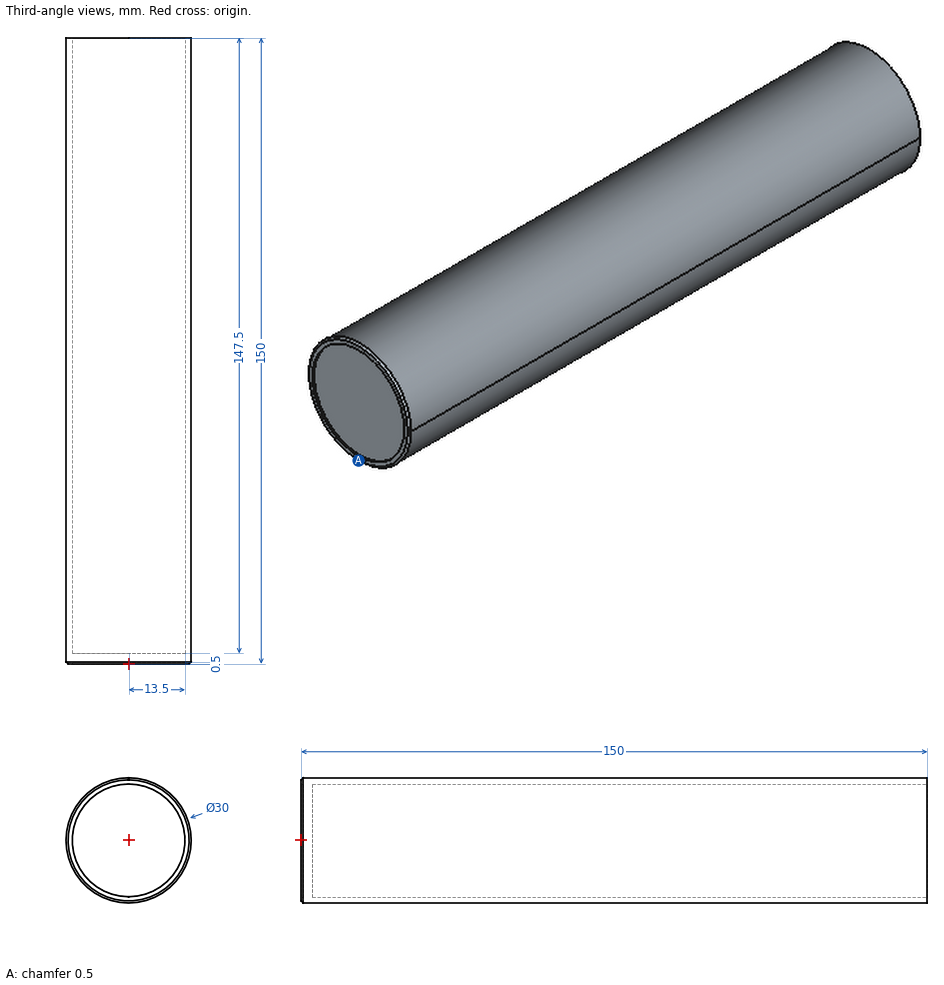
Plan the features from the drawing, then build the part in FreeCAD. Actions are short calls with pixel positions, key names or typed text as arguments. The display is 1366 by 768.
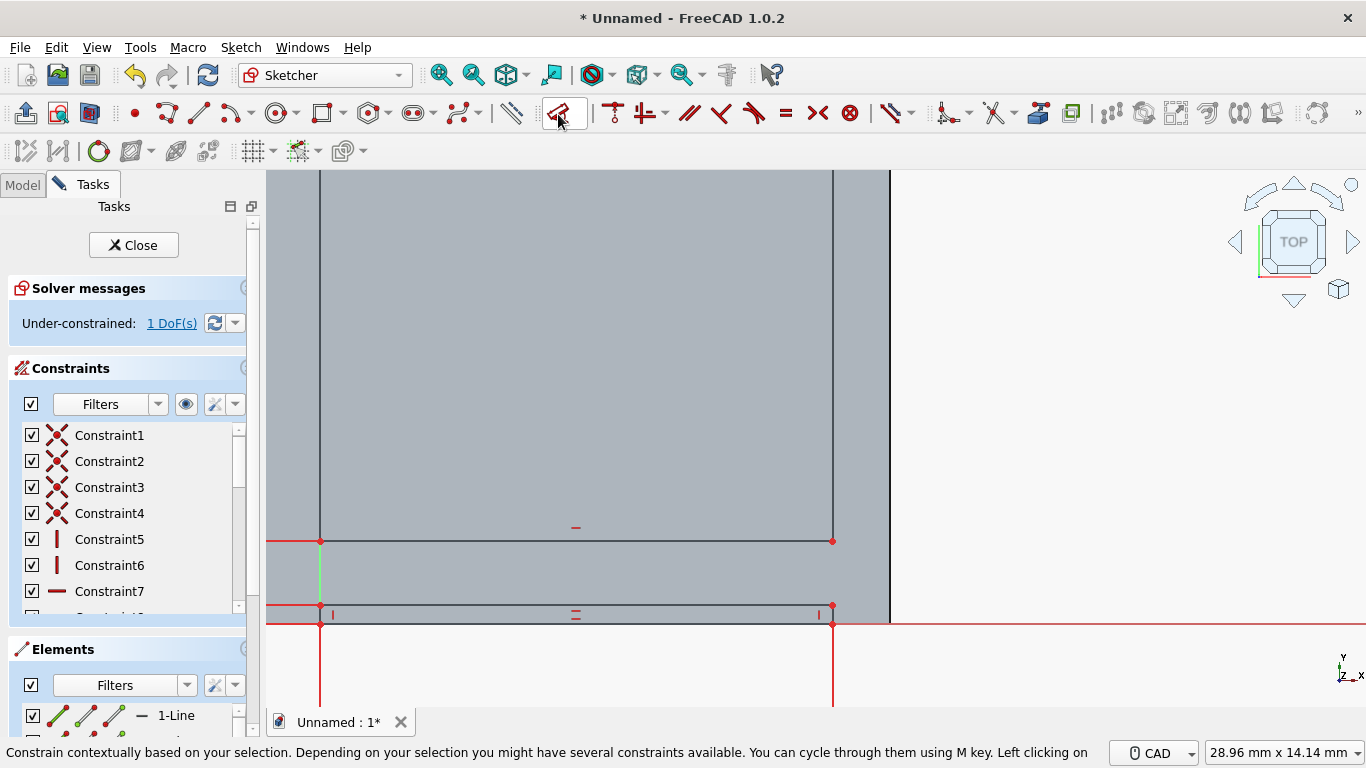
scroll(759, 611, down, 14)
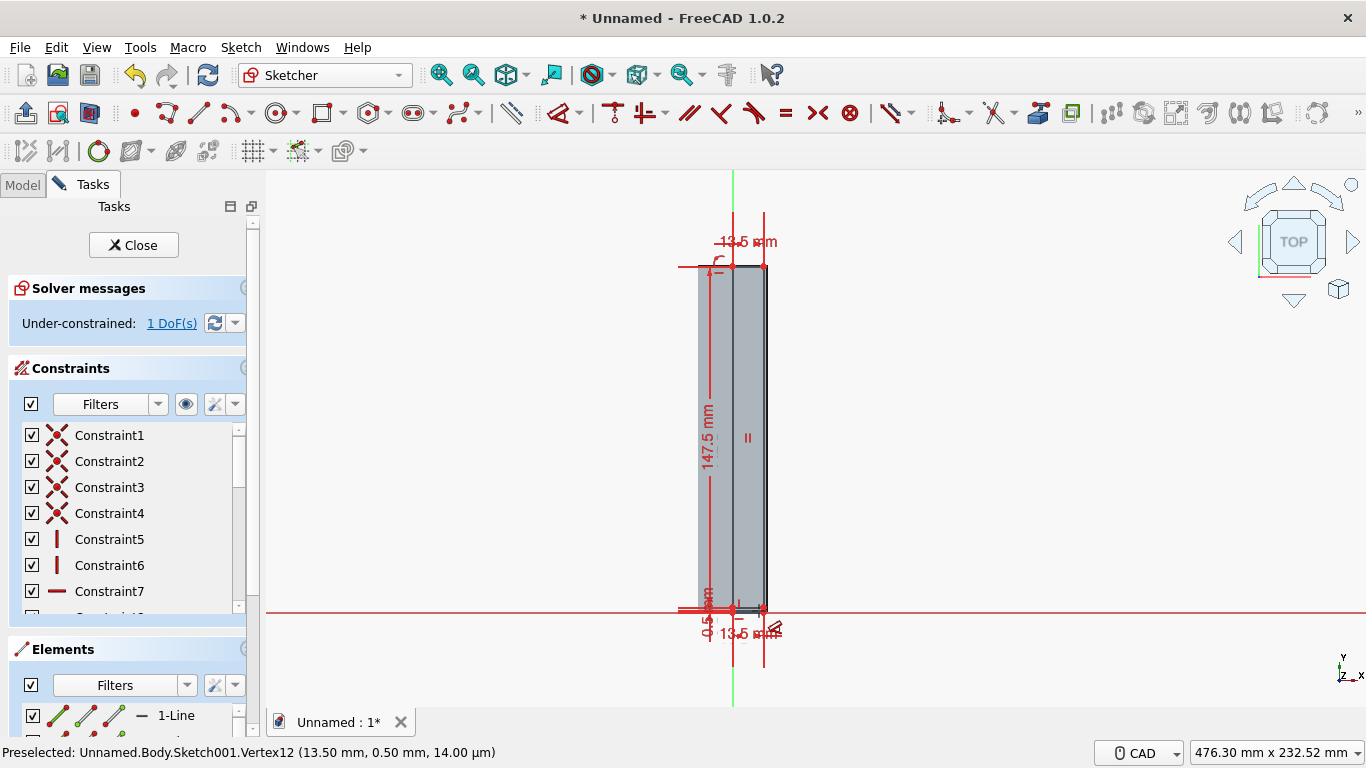
click(733, 267)
click(699, 440)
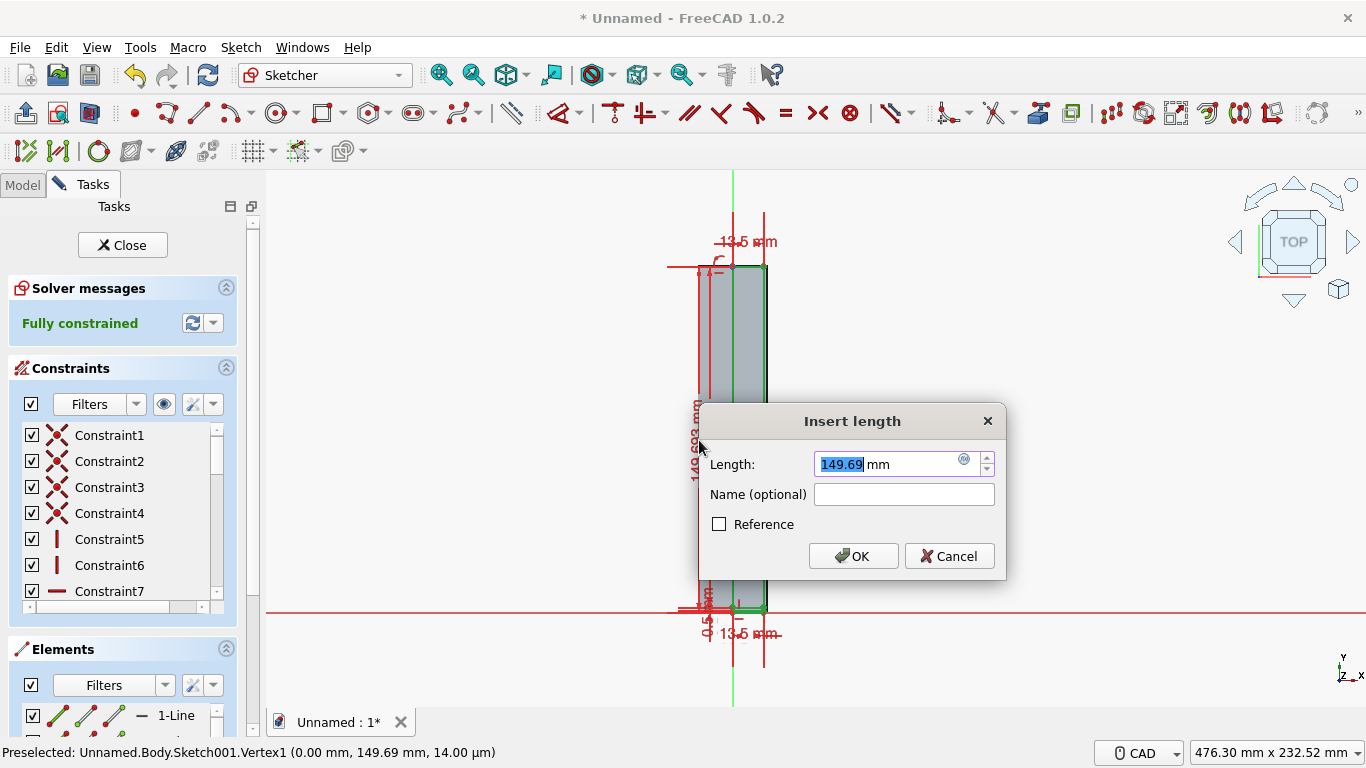
text(150)
key(Return)
key(Escape)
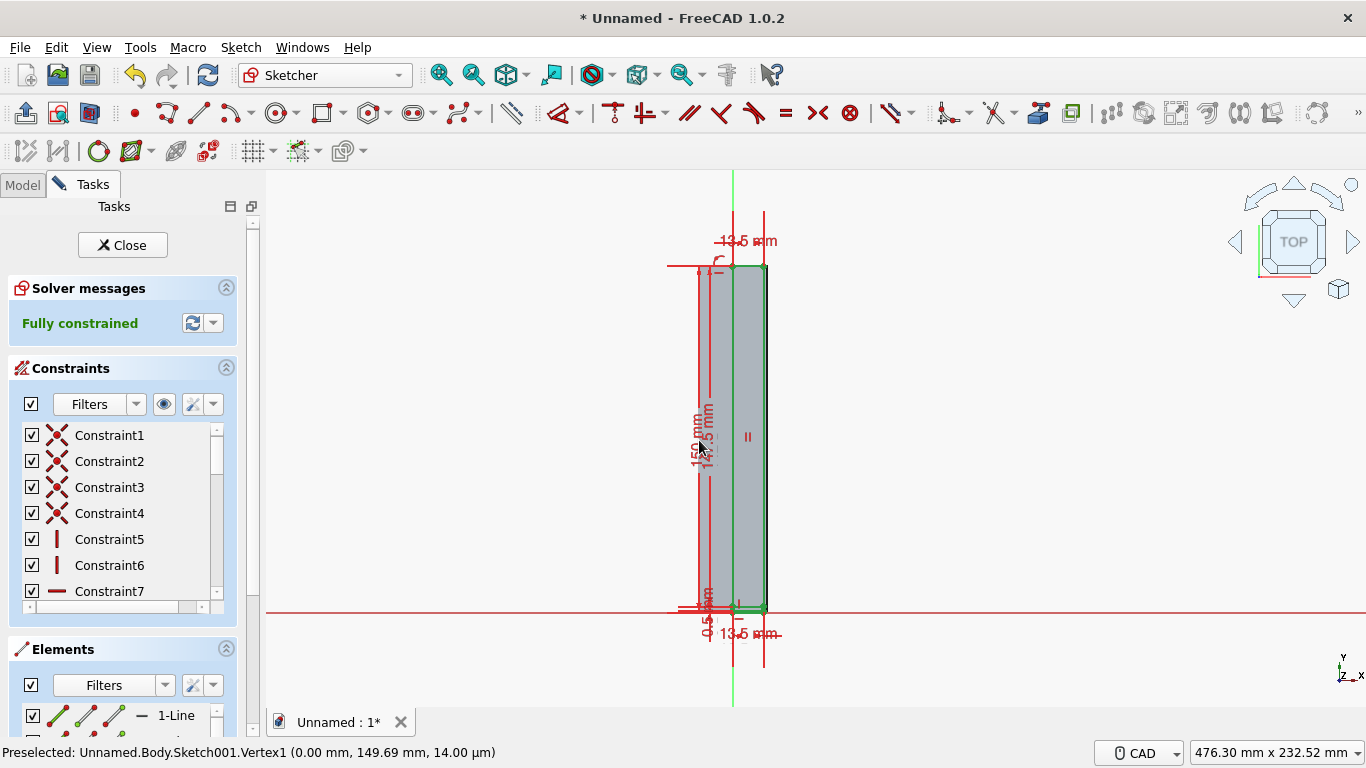
click(123, 245)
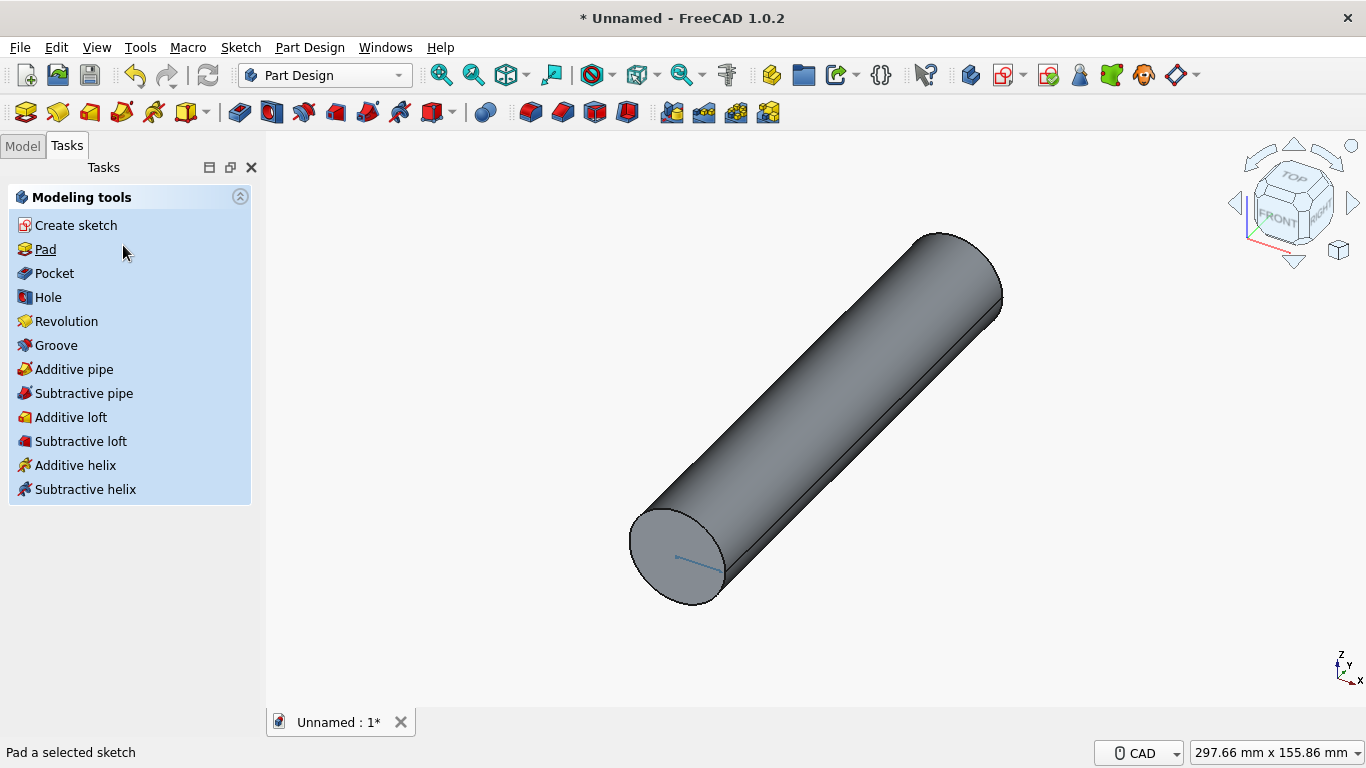
click(304, 112)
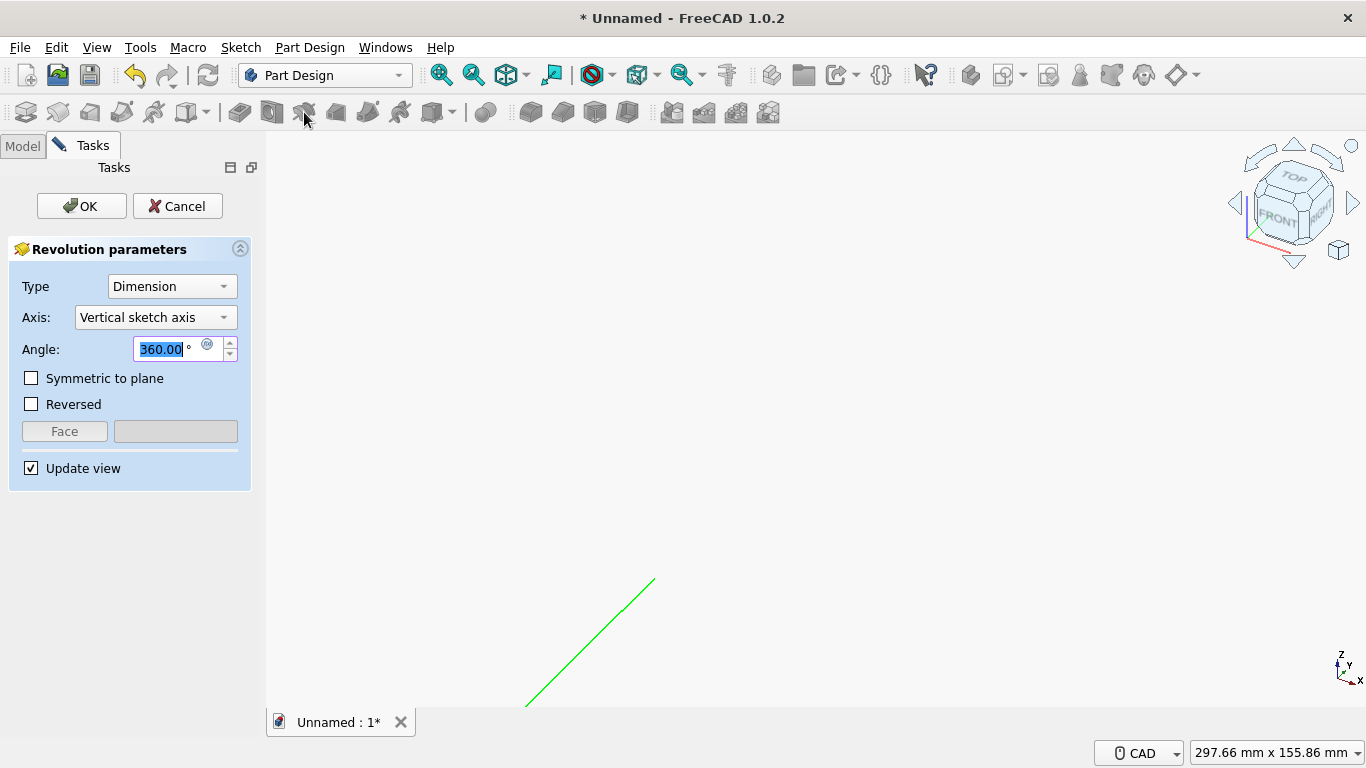
click(82, 206)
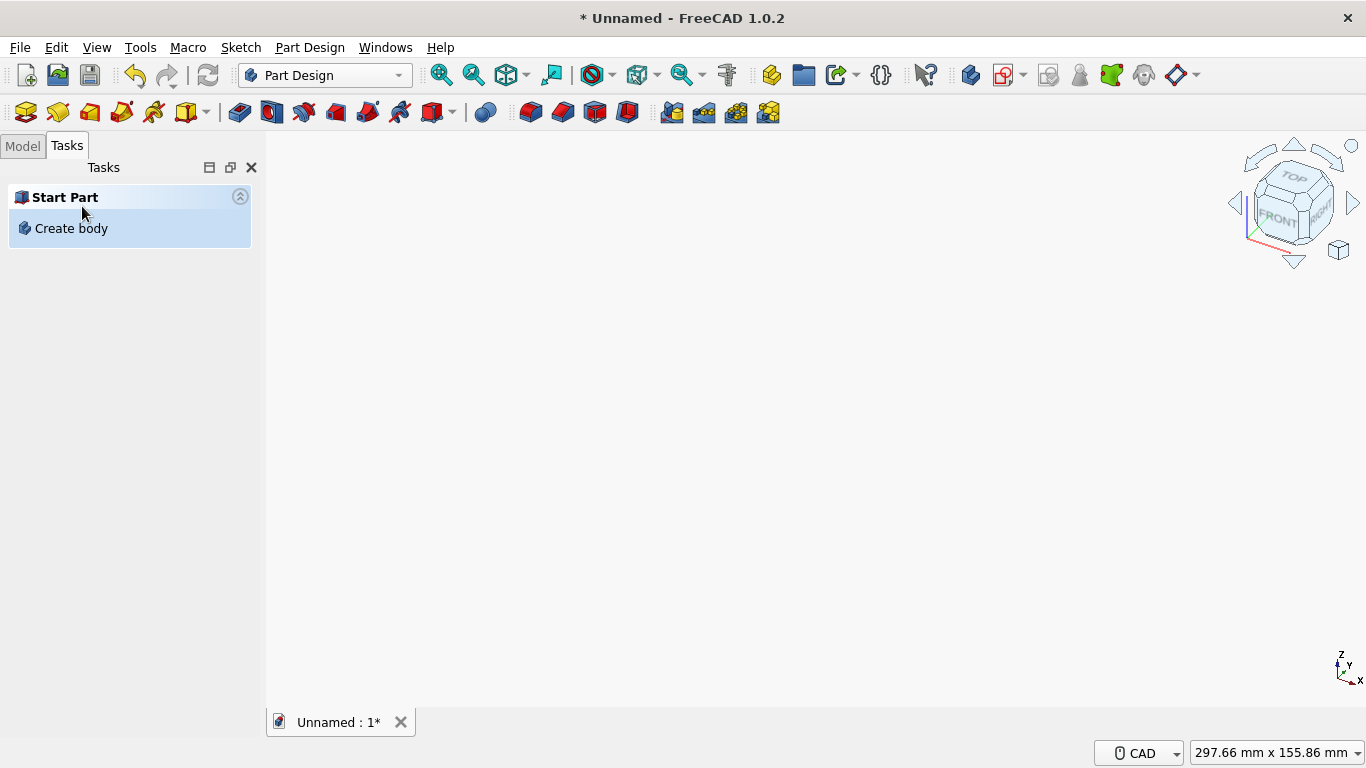
click(442, 76)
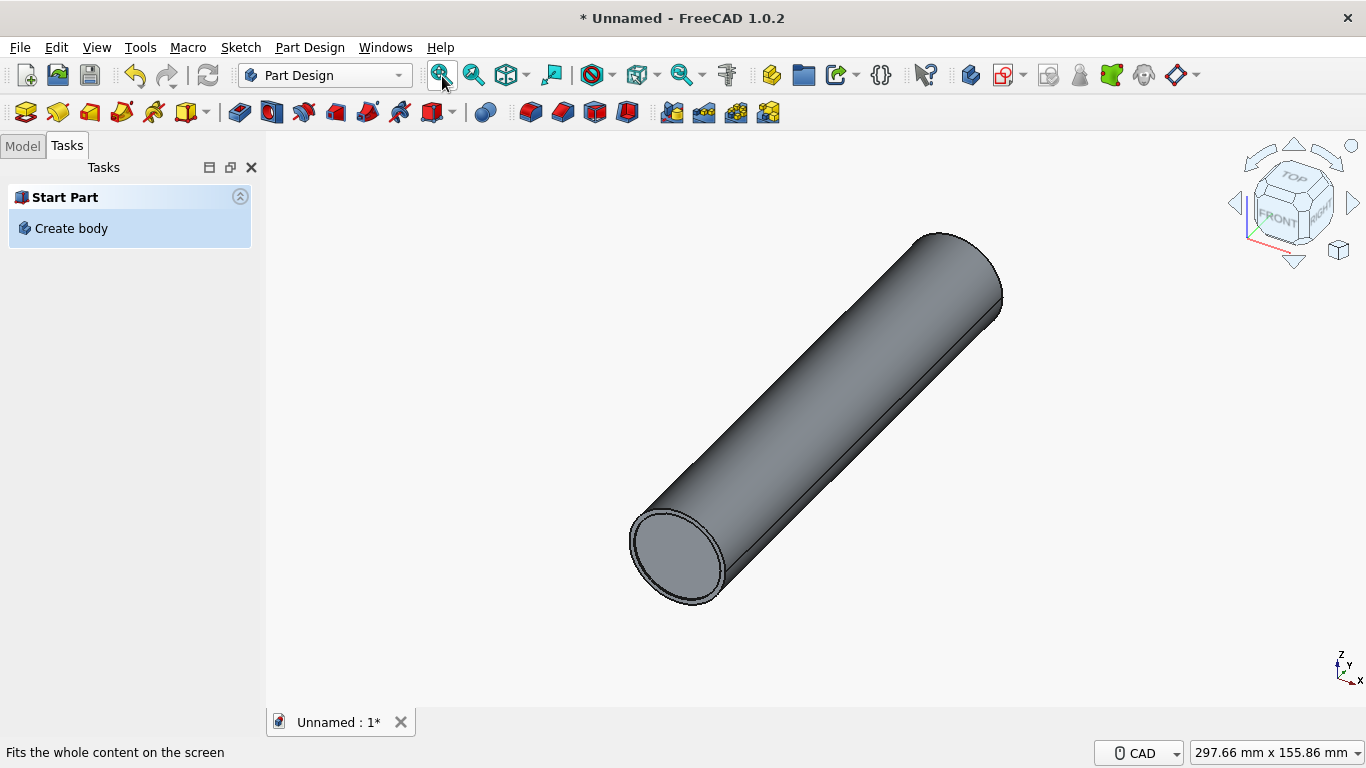
click(638, 516)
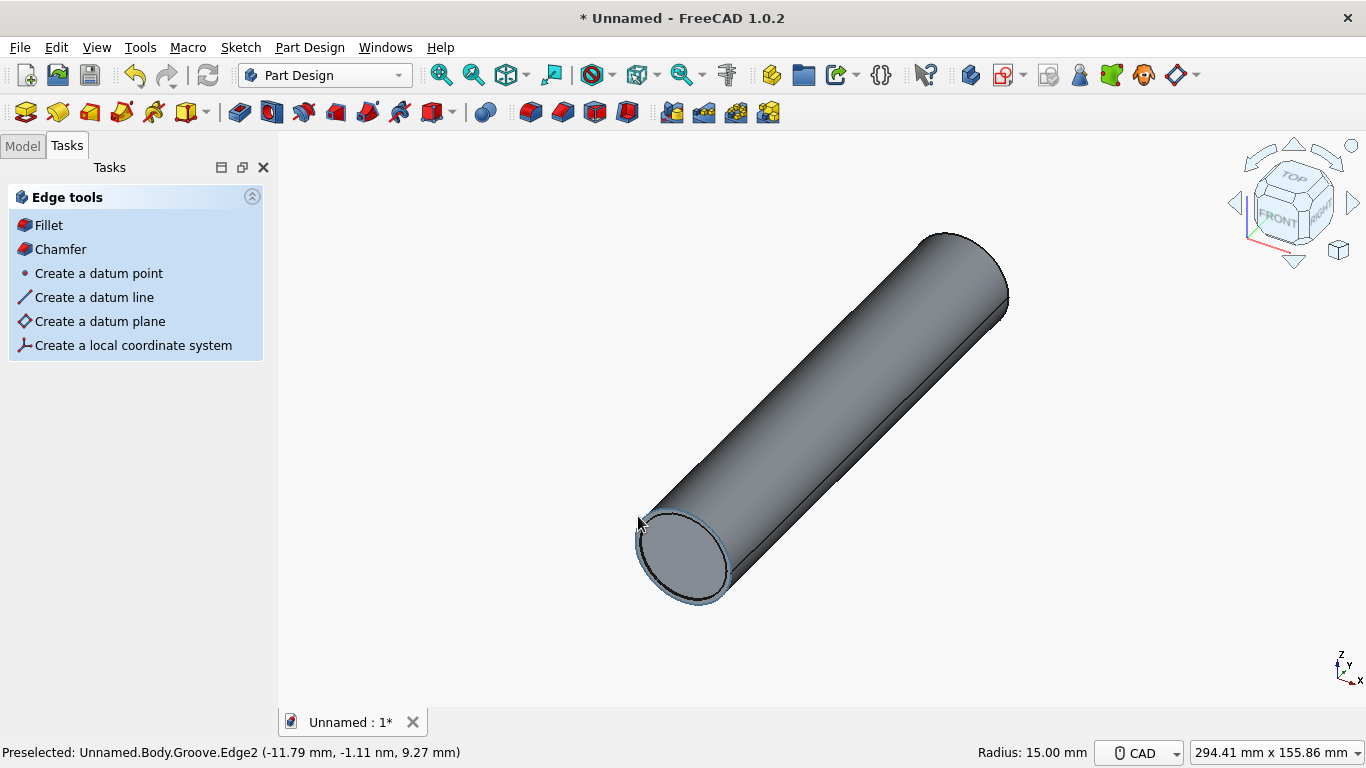
click(564, 112)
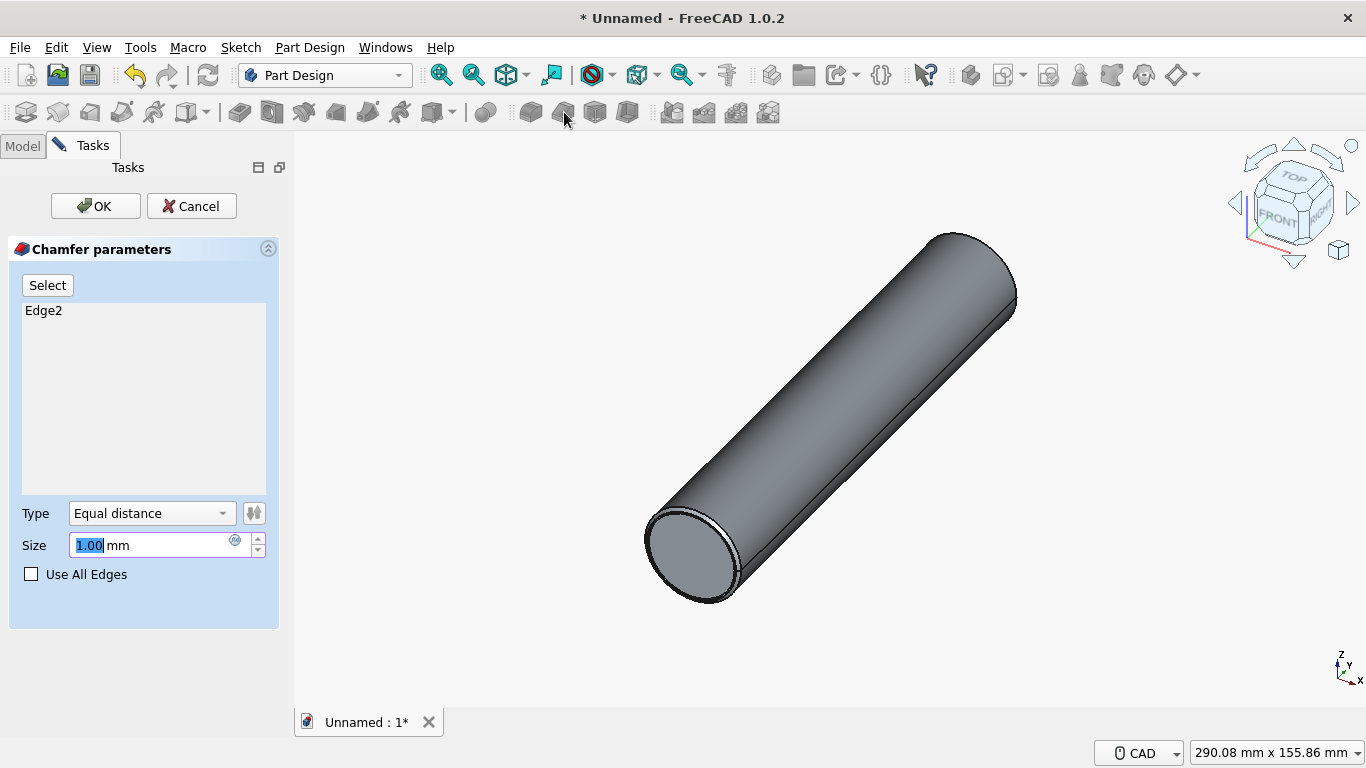
text(0.5)
key(Tab)